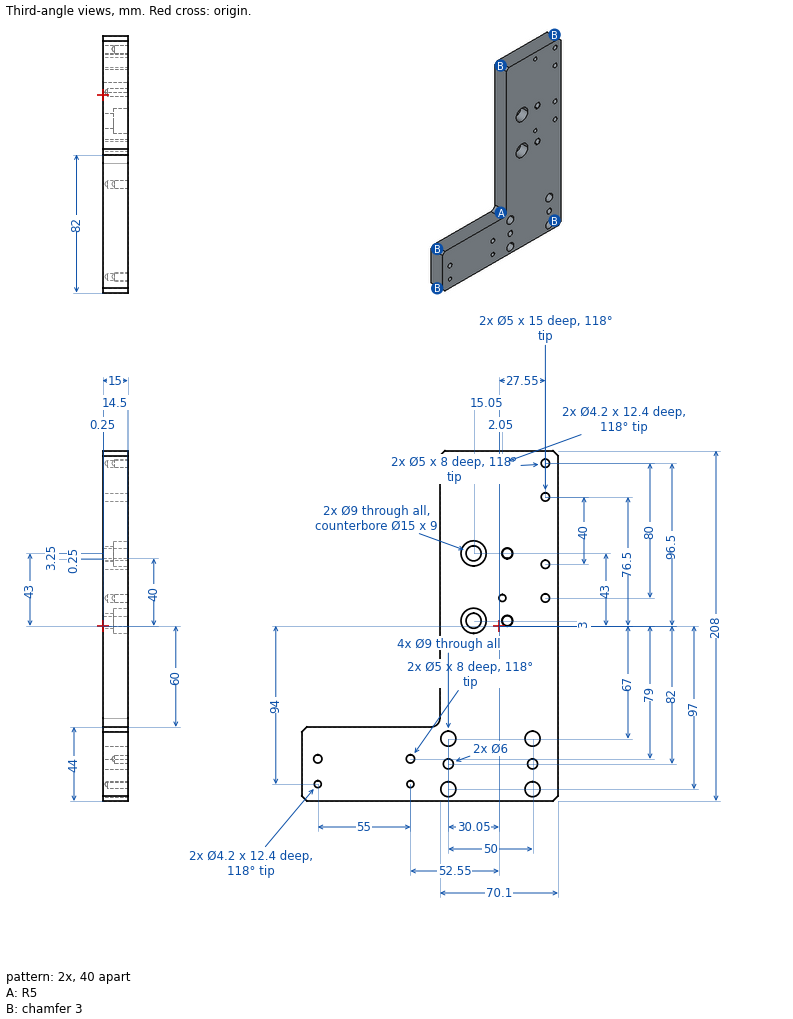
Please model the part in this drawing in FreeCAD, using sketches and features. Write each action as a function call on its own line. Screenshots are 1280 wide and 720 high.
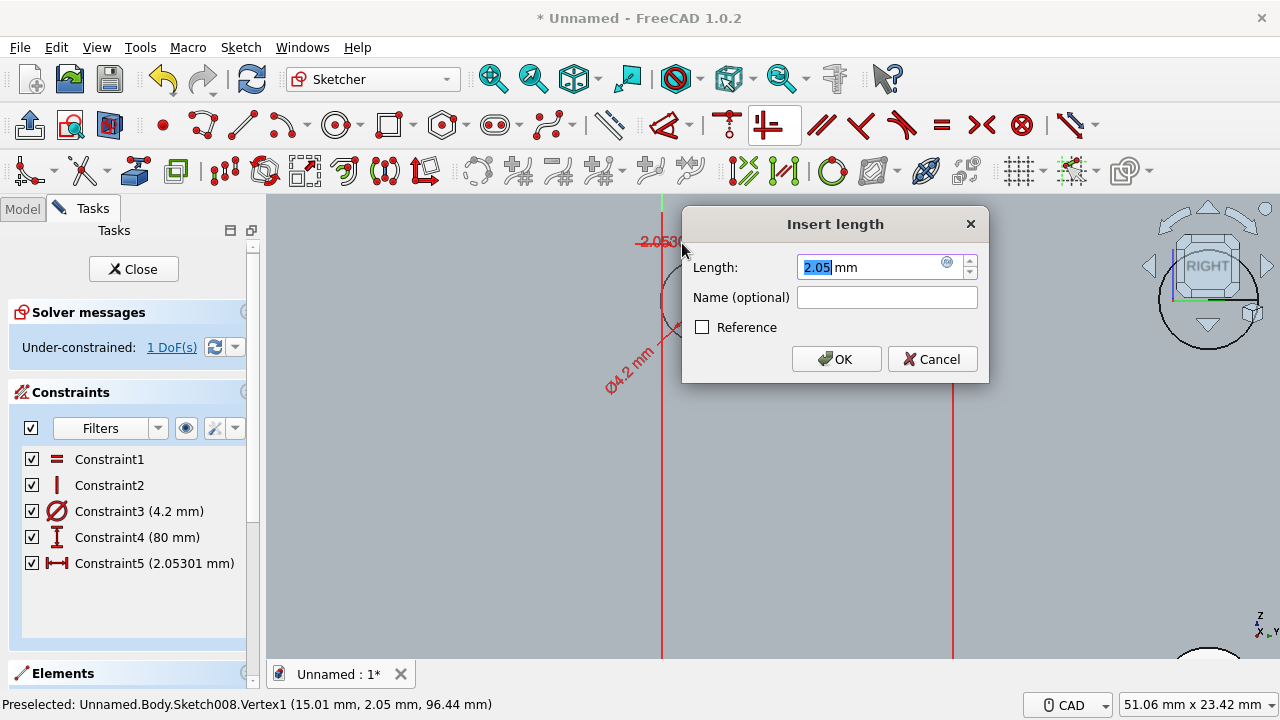
text(2.05)
key(Return)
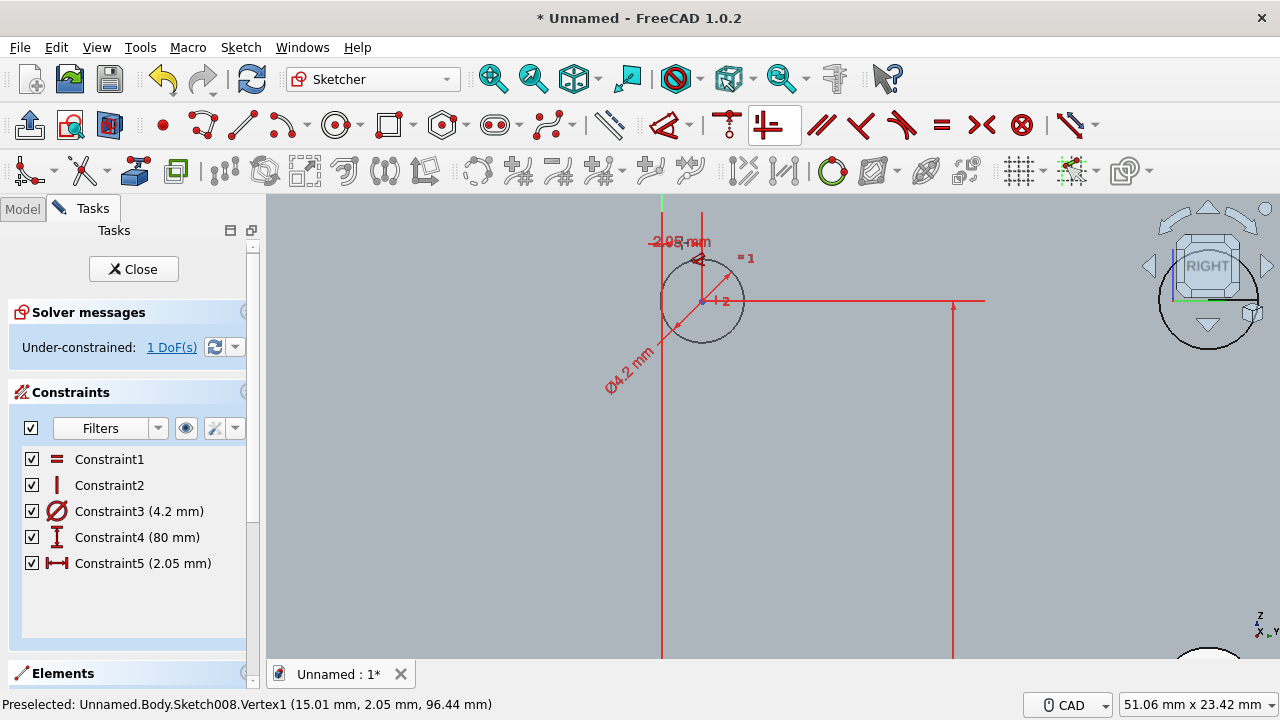
scroll(705, 300, down, 10)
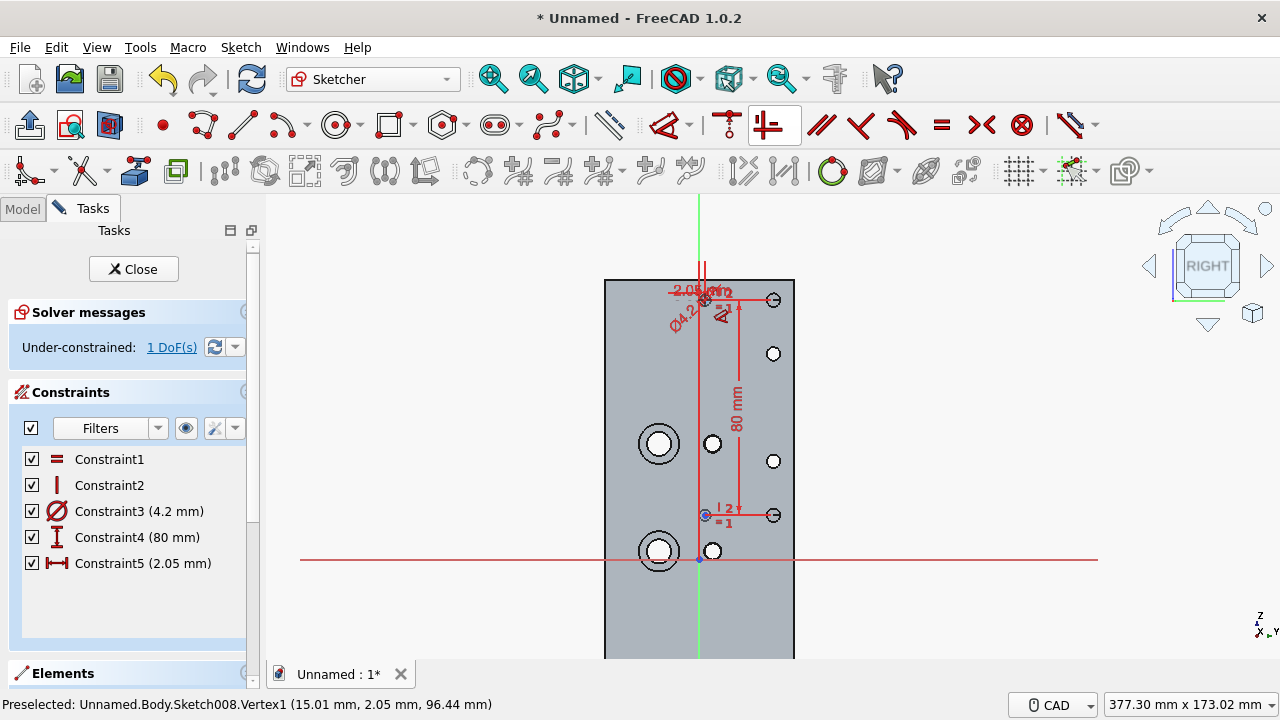
click(705, 300)
click(665, 430)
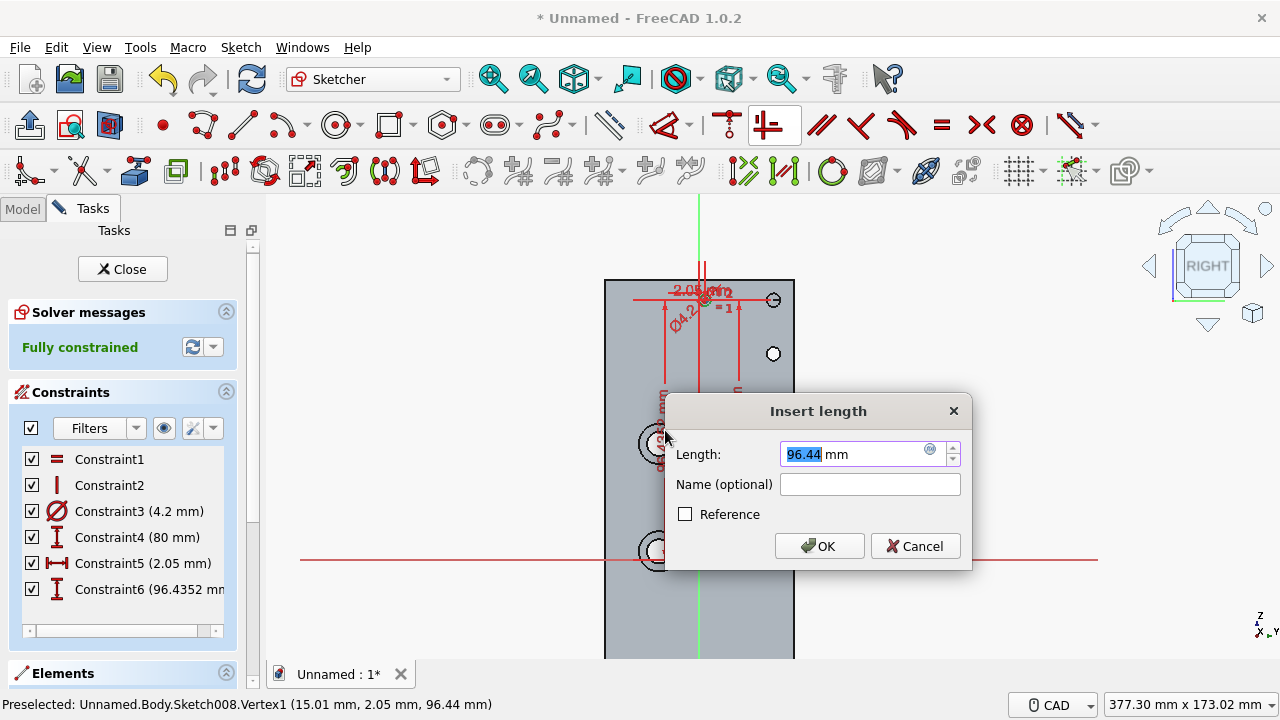
text(96.5)
key(Return)
key(Escape)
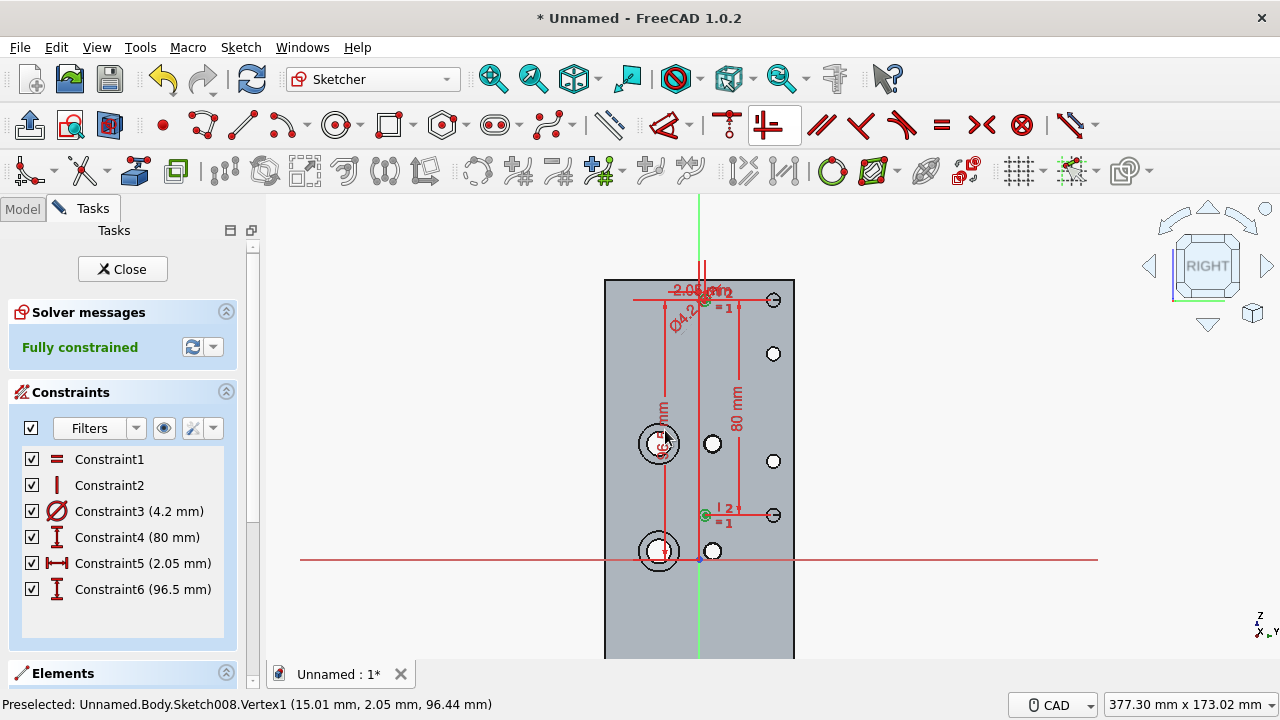
click(123, 269)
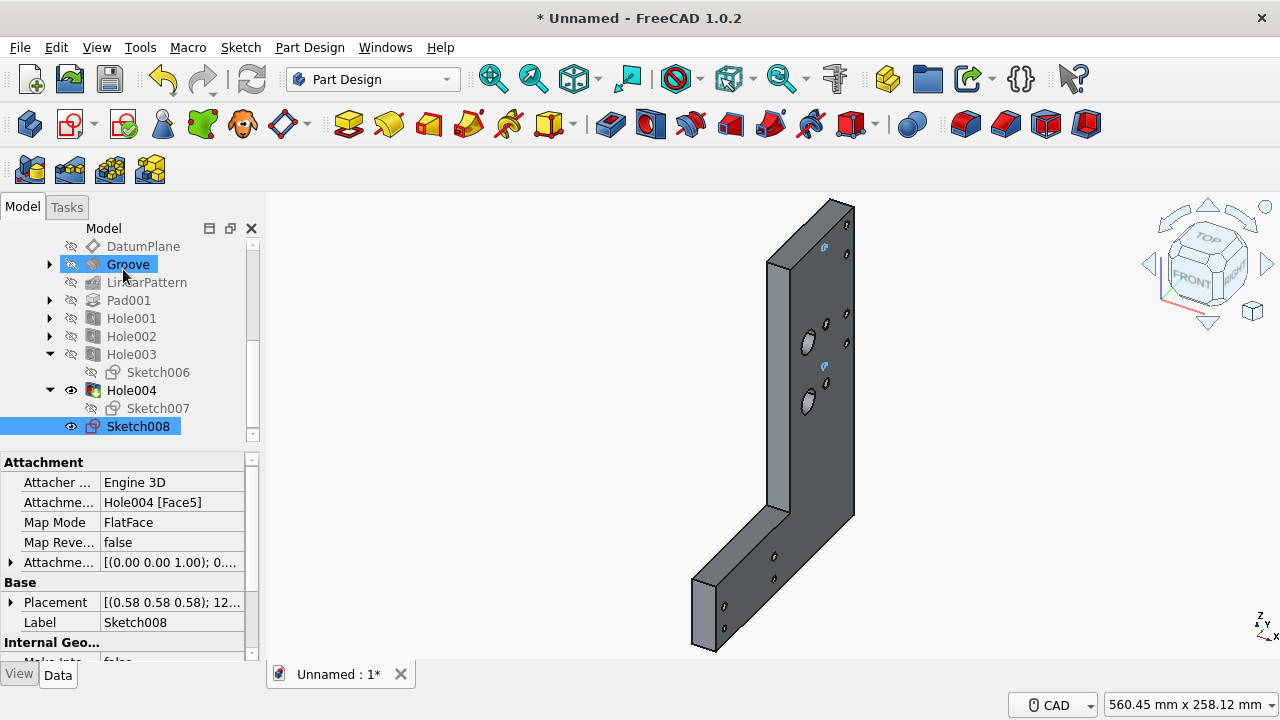
click(652, 124)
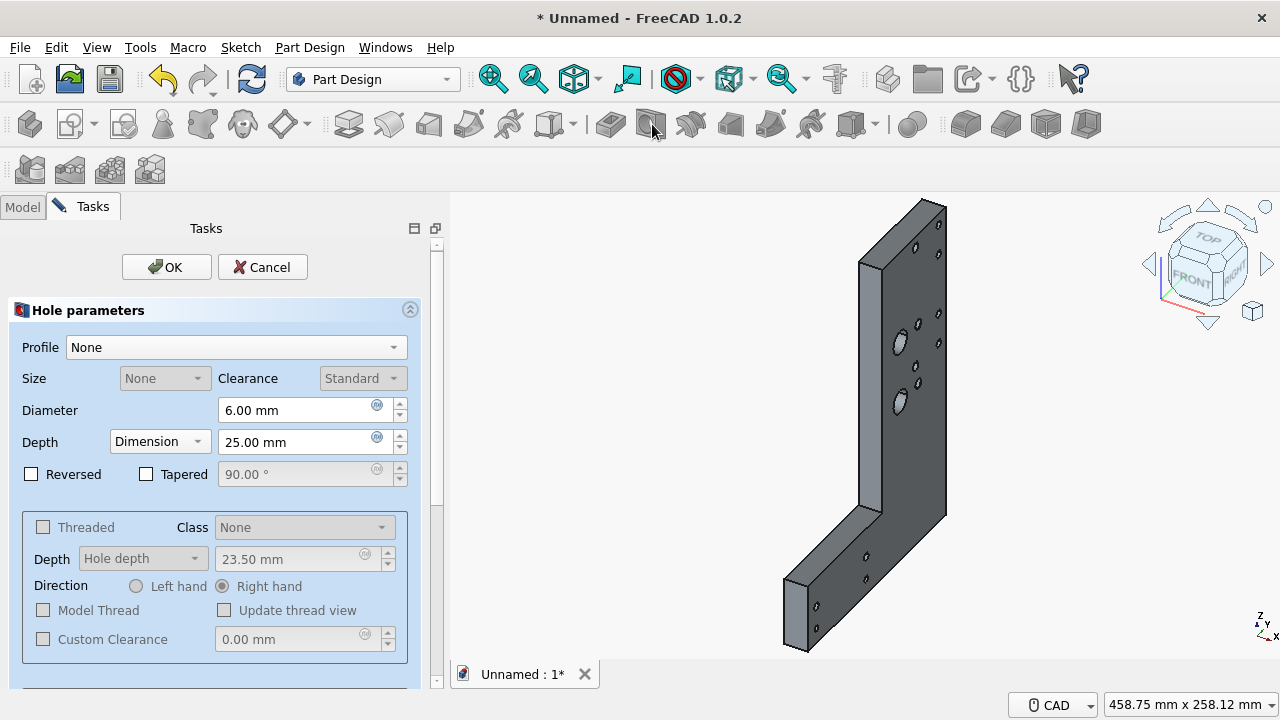
triple_click(305, 410)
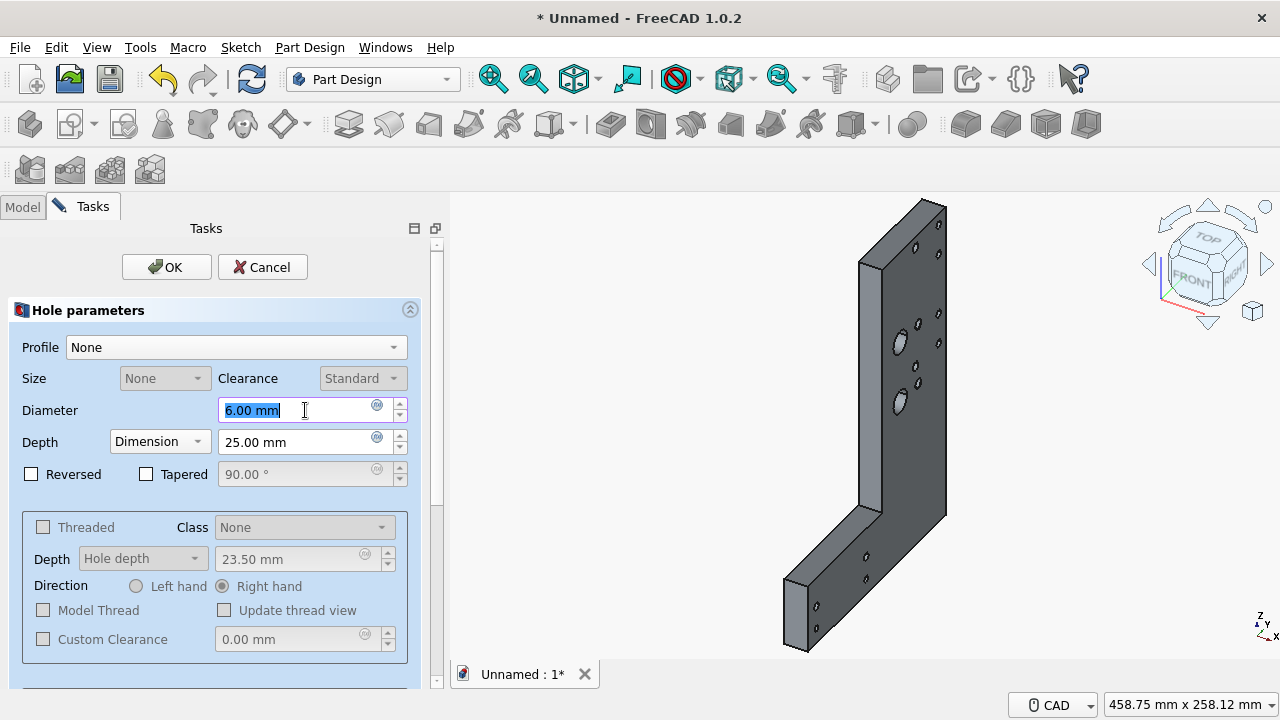
text(4.2)
key(Tab)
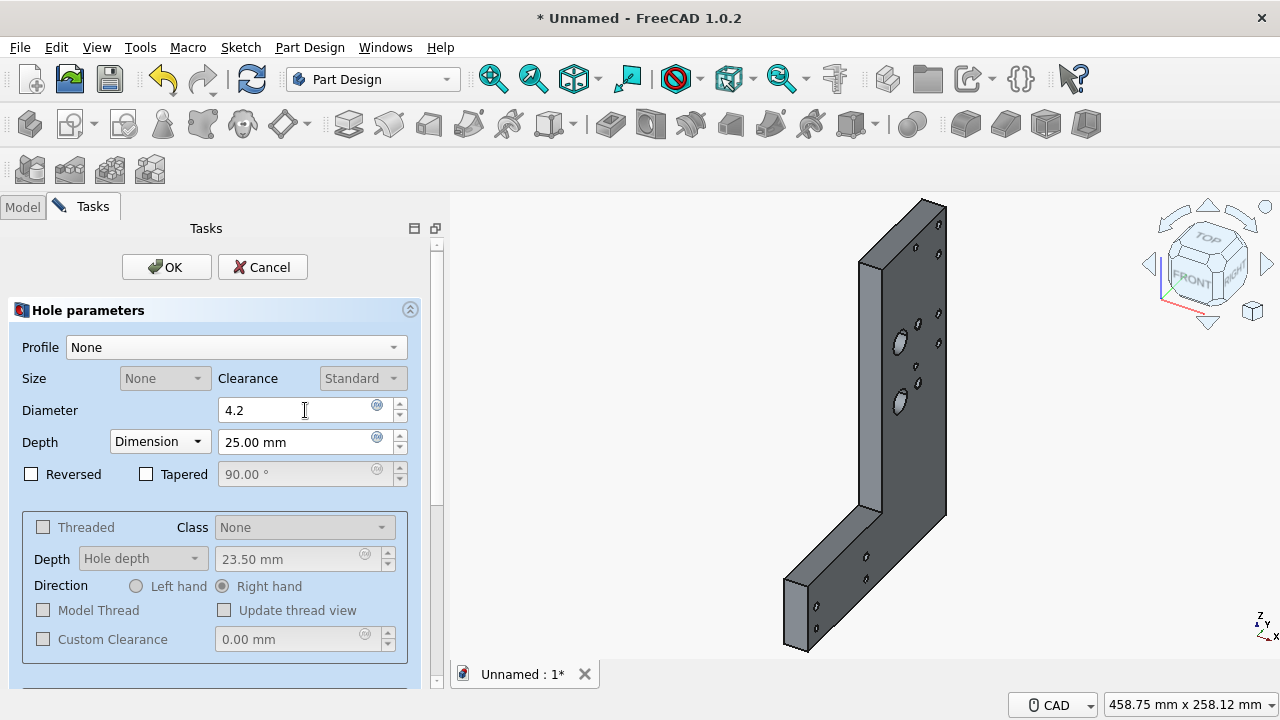
triple_click(305, 442)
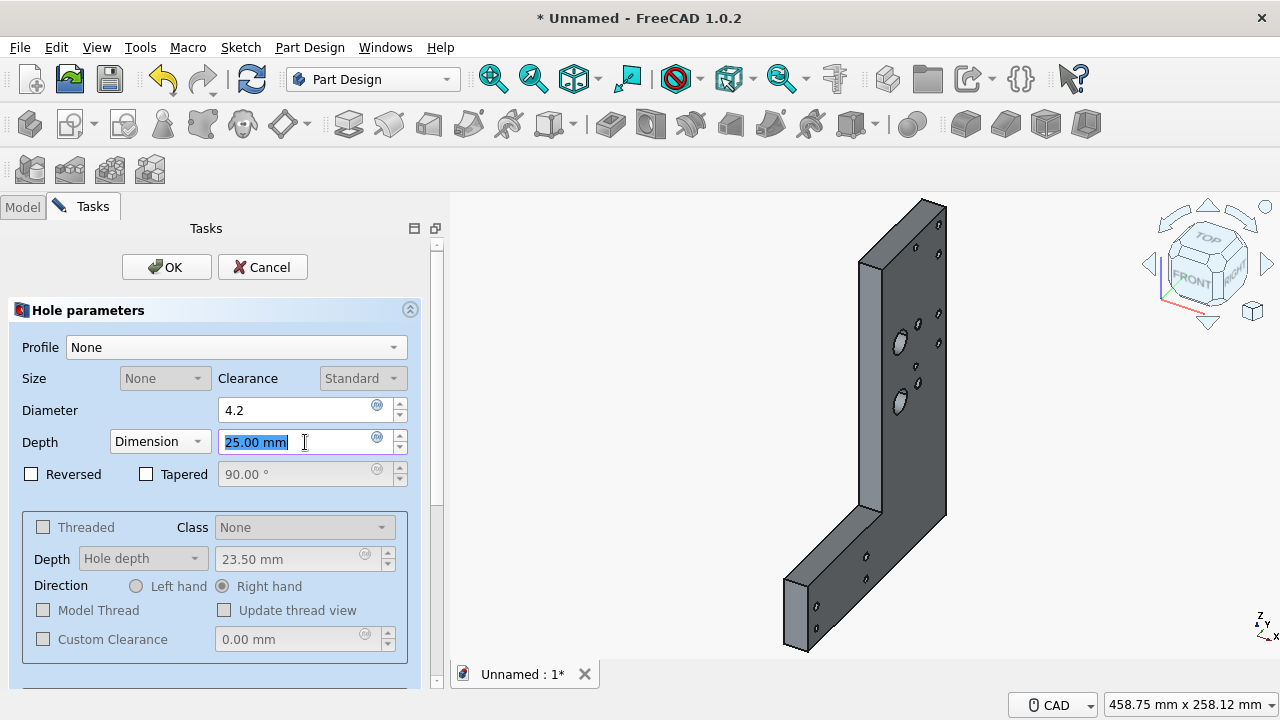
text(12.4)
key(Tab)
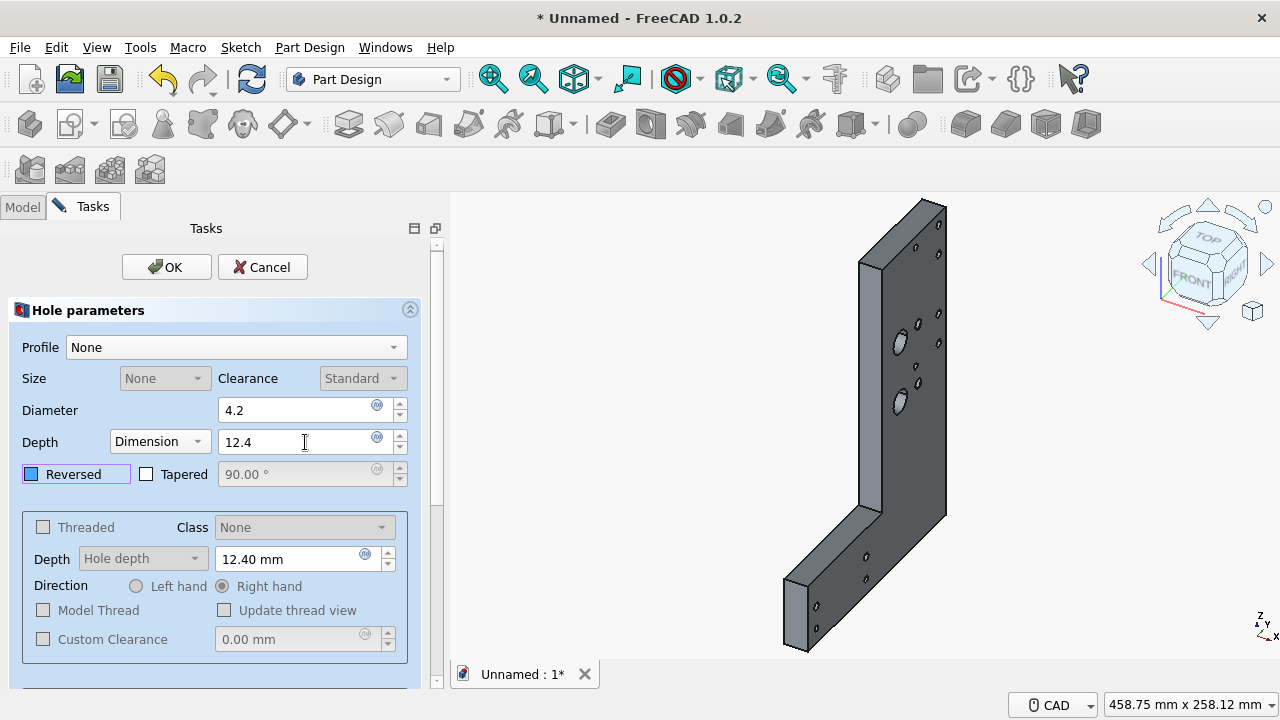
click(167, 267)